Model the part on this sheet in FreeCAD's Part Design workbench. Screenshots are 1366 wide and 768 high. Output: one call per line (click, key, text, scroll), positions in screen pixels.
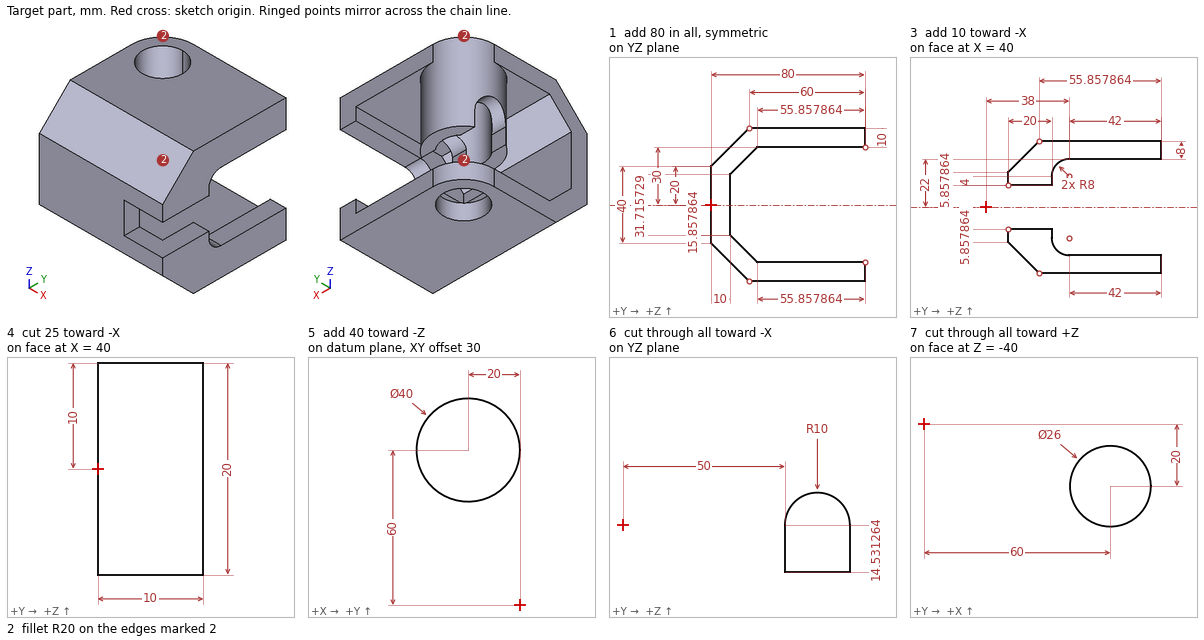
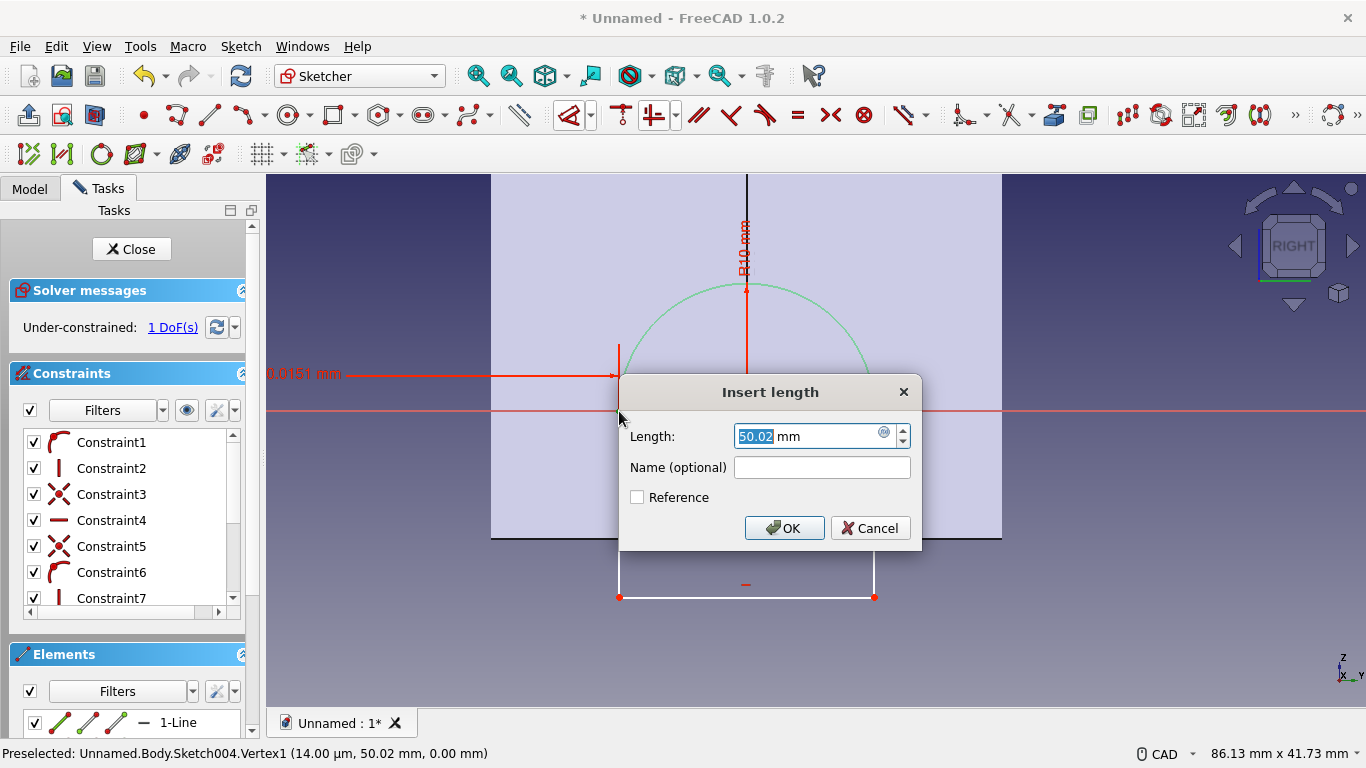
text(50)
key(Return)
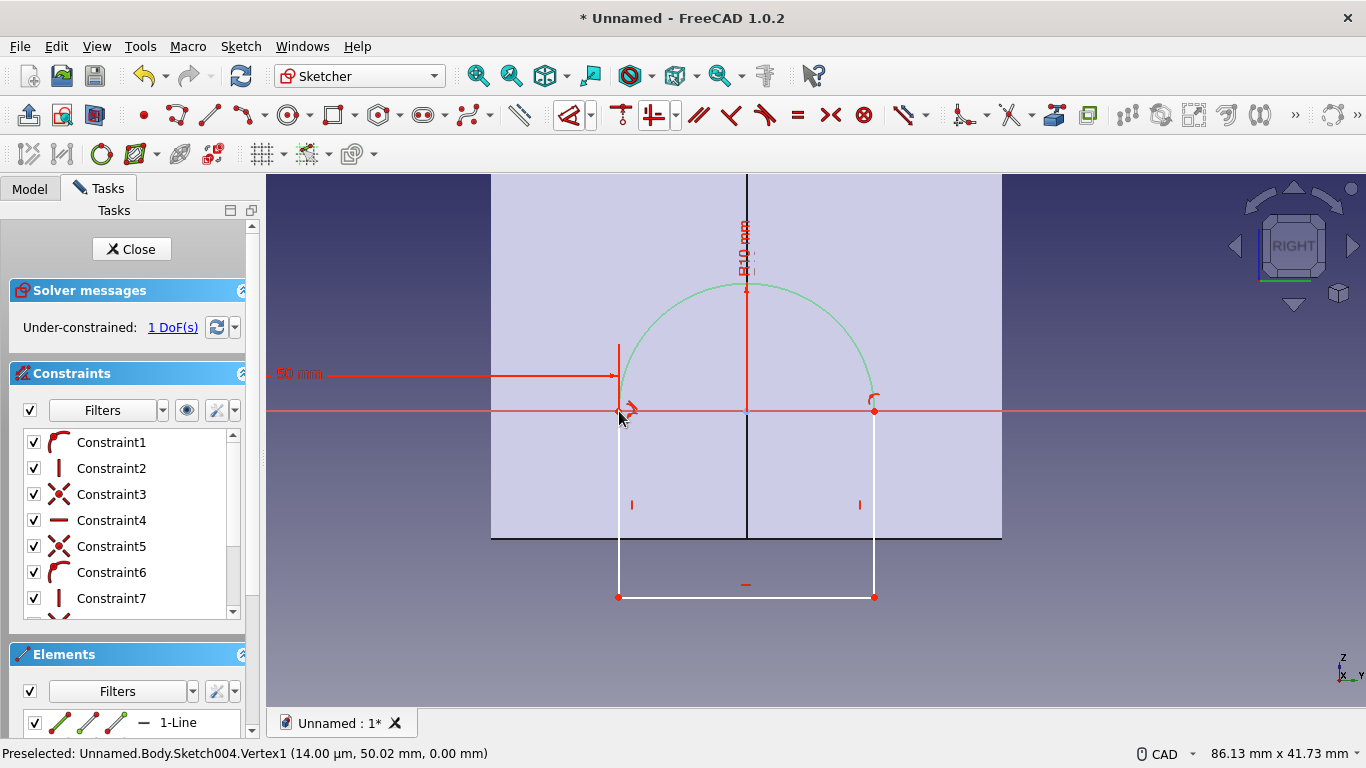
click(619, 467)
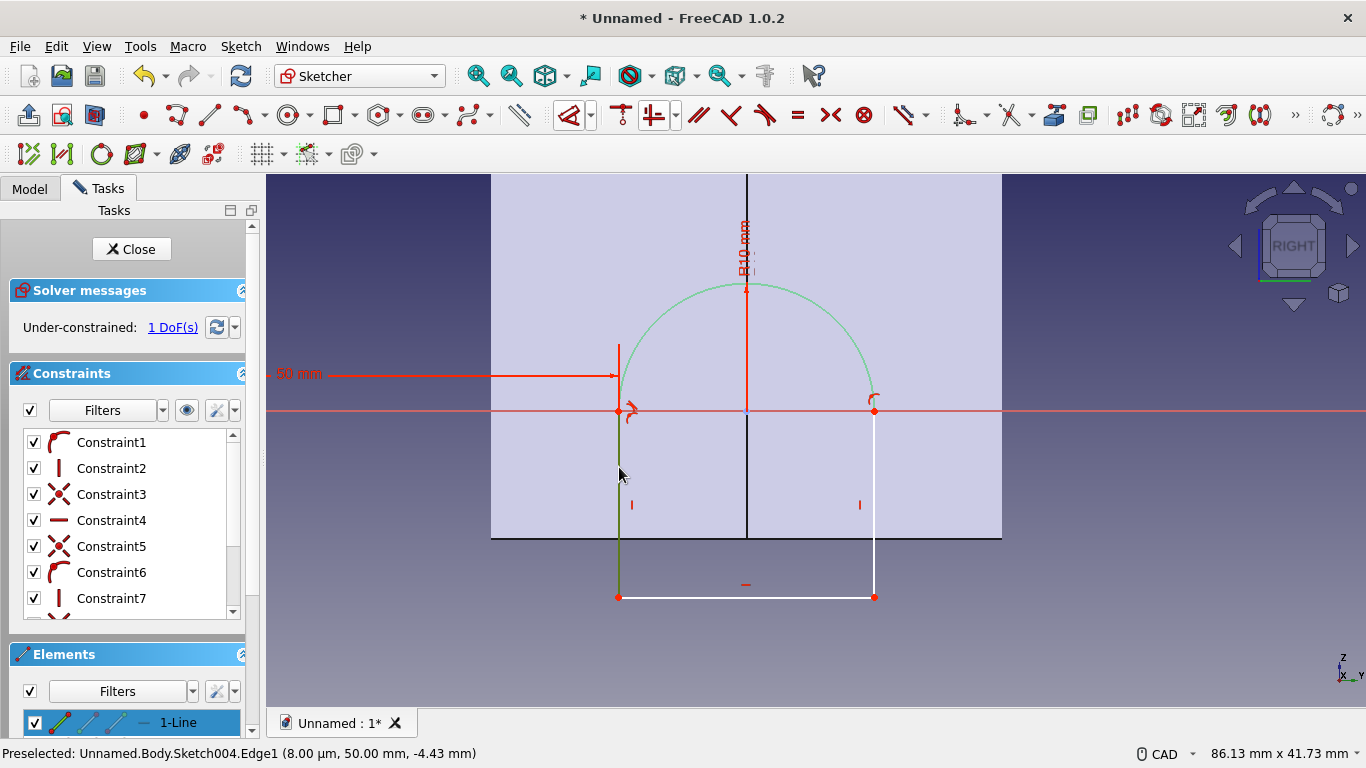
click(590, 116)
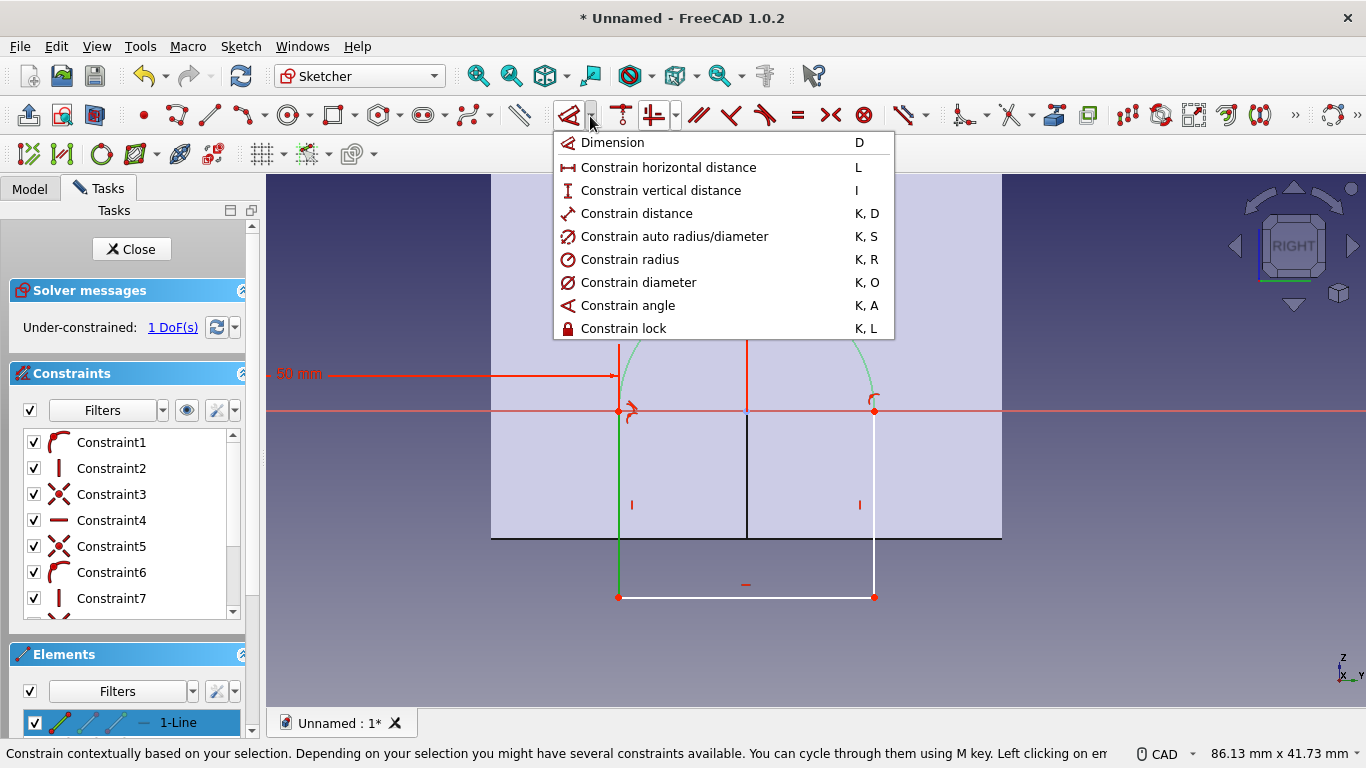
click(724, 190)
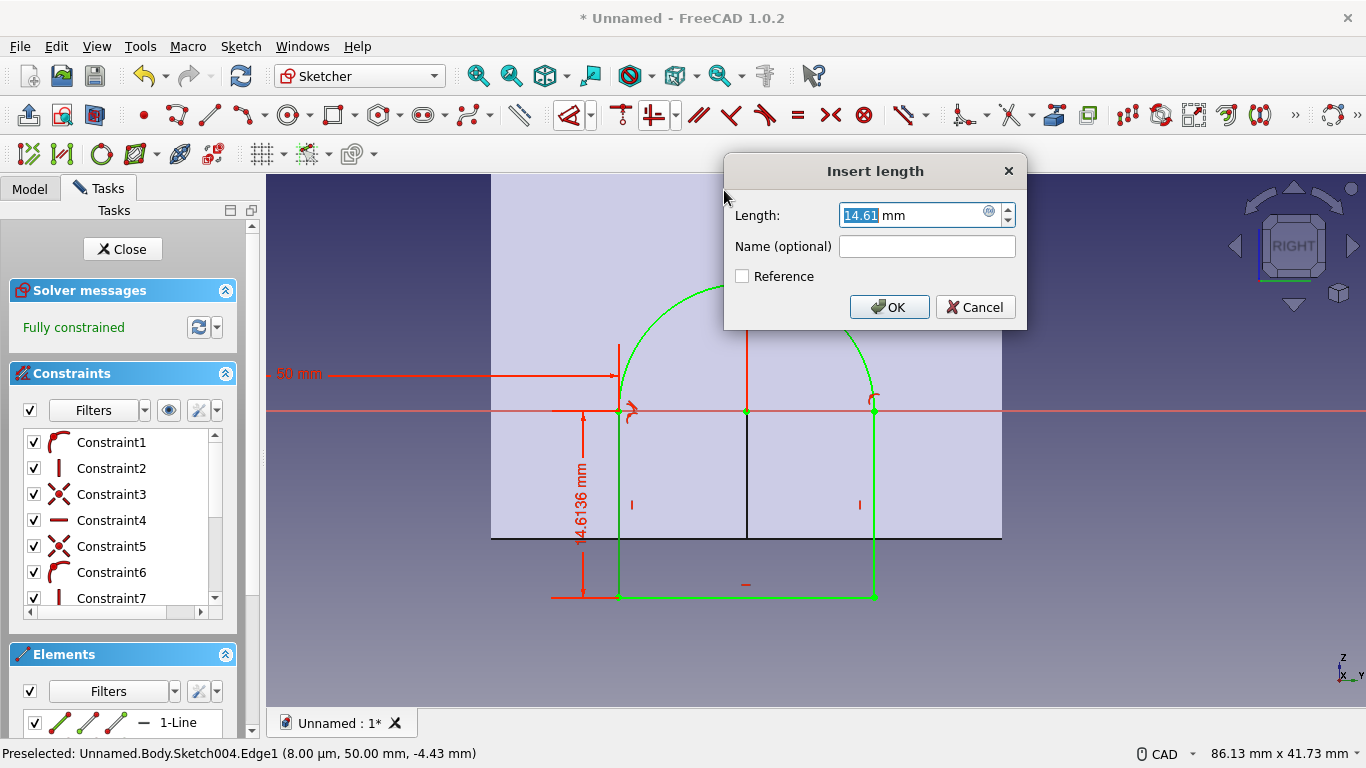
text(14.531264)
key(Return)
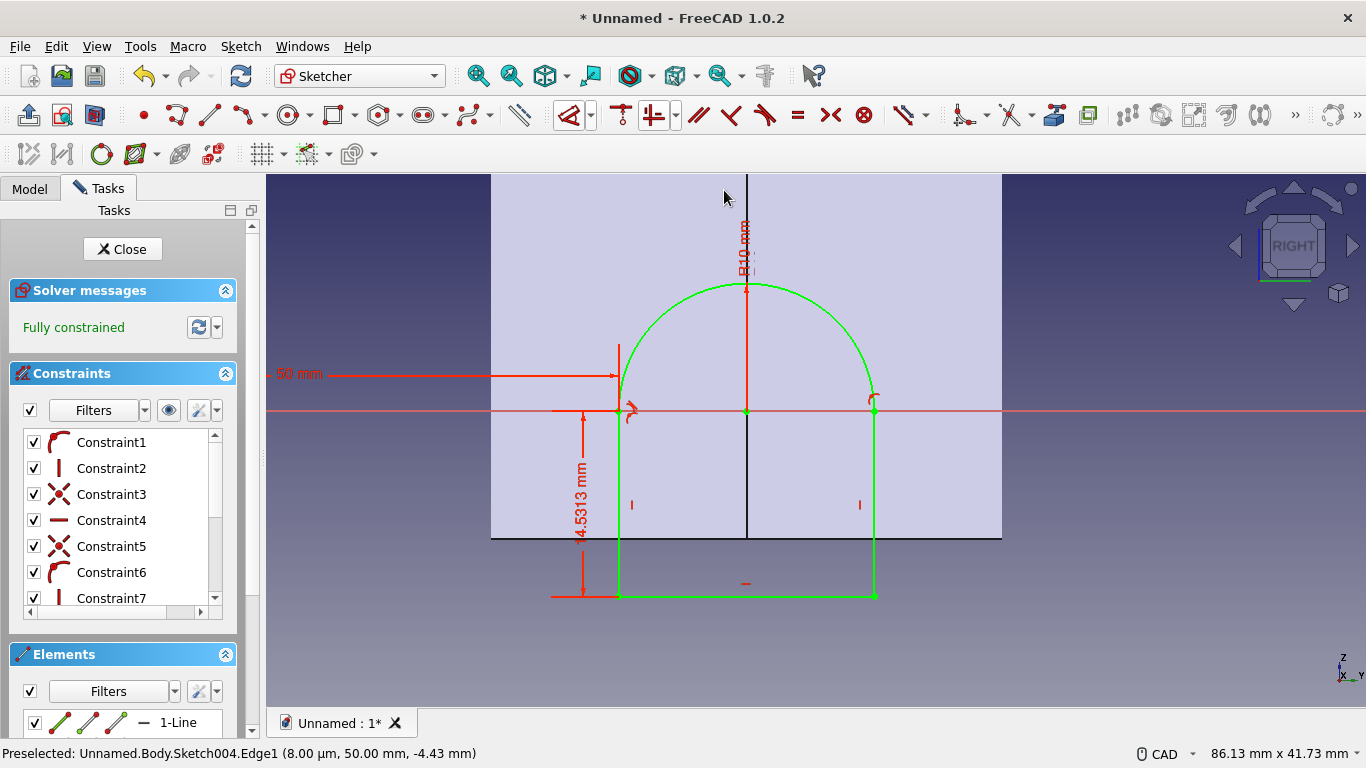
click(123, 249)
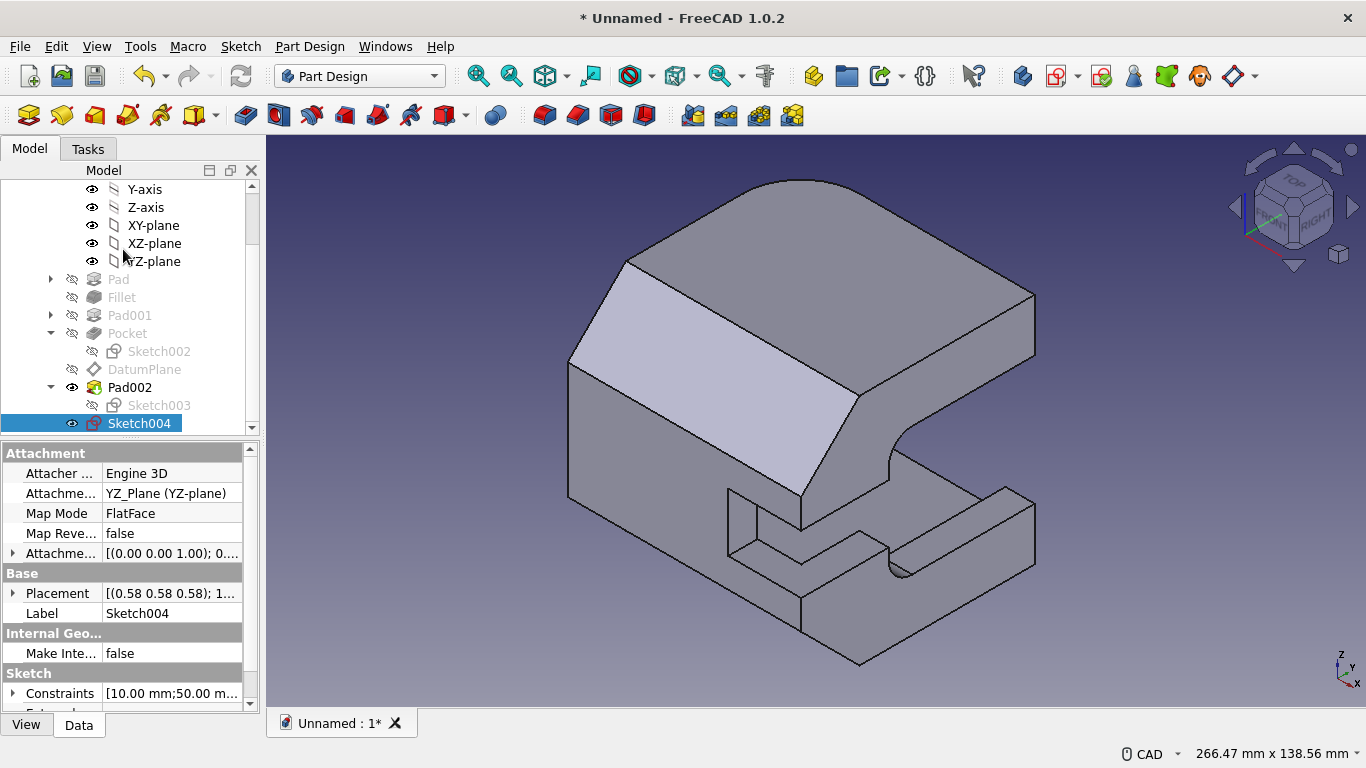
click(246, 116)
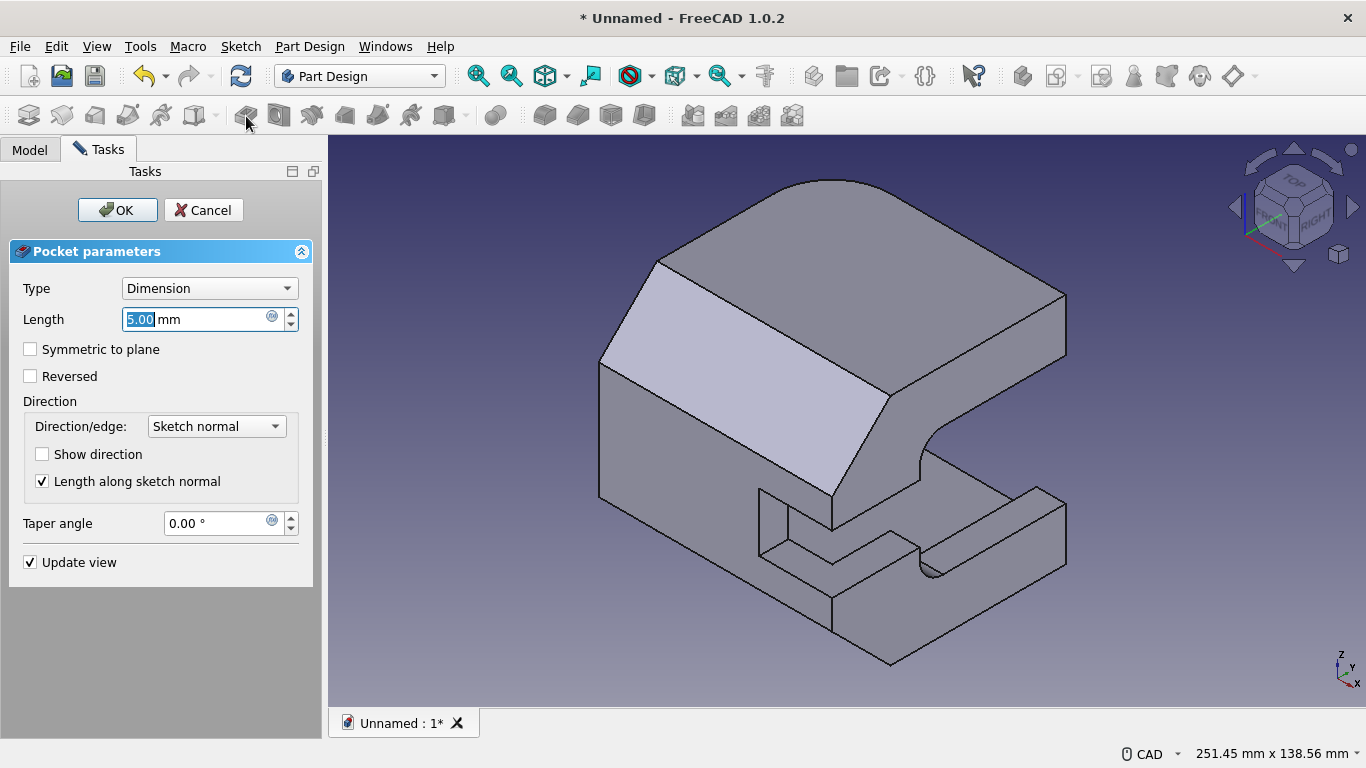
click(210, 288)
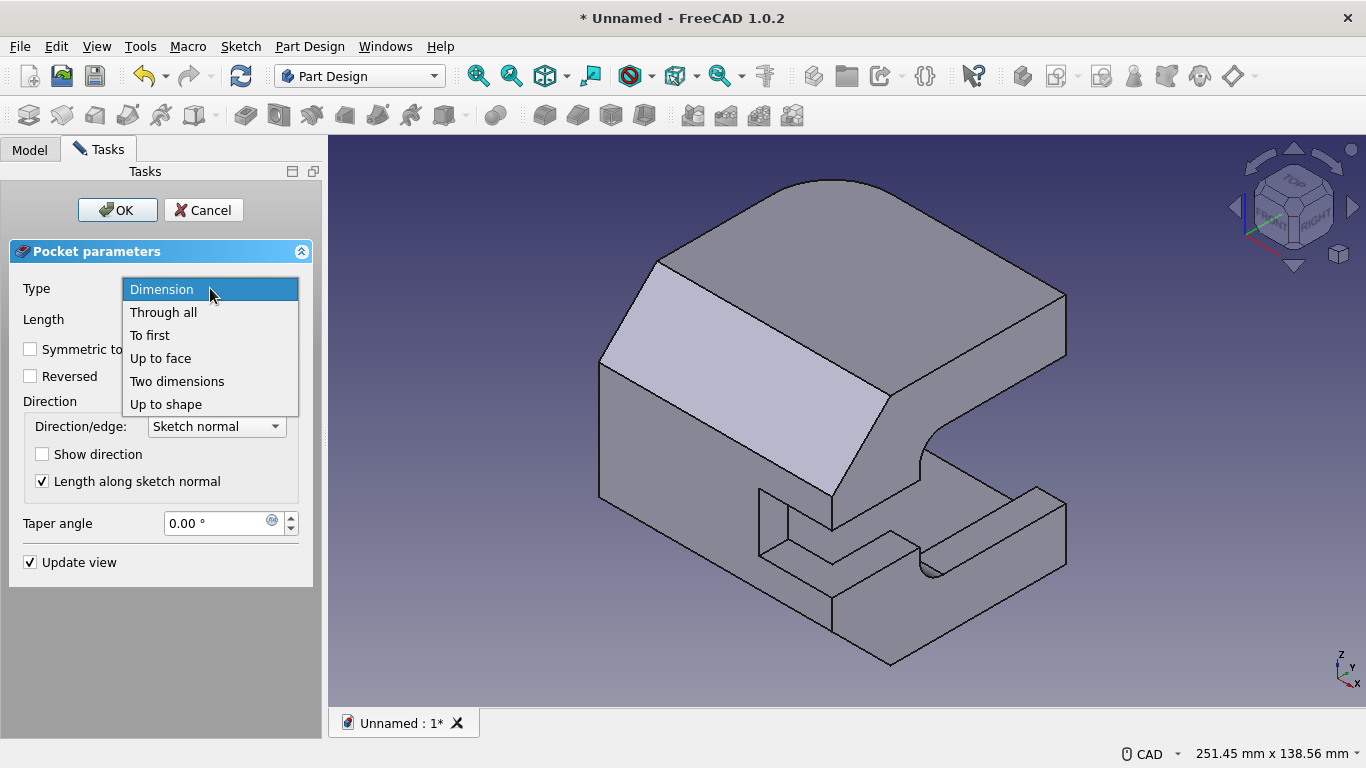
click(208, 312)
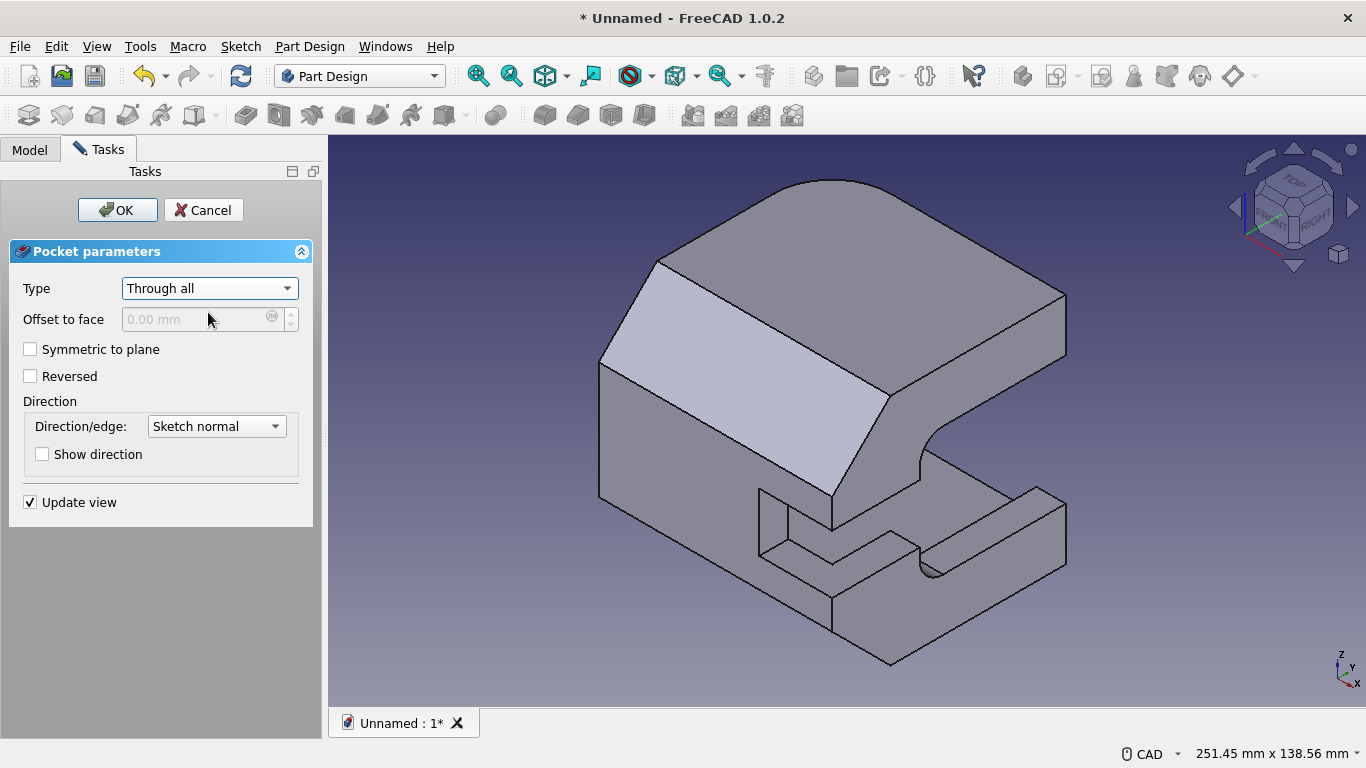
click(118, 210)